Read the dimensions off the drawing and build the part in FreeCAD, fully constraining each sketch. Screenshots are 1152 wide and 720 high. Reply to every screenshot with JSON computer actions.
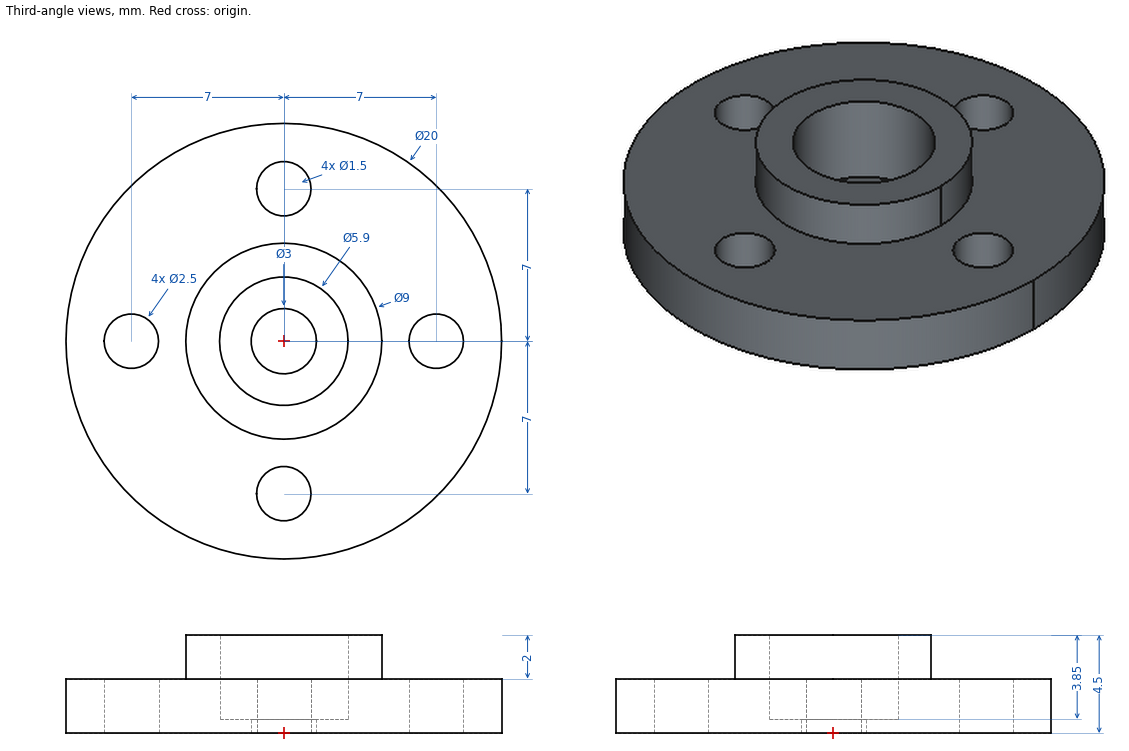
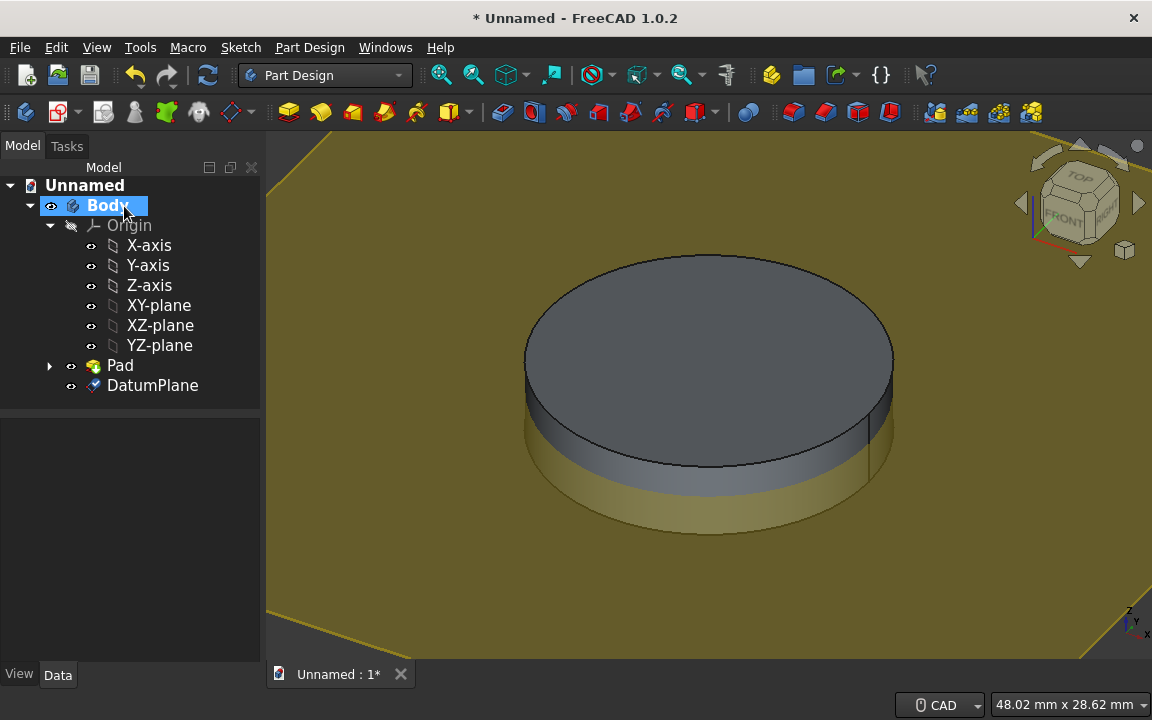
{"action": "left_click", "coordinate": [116, 386]}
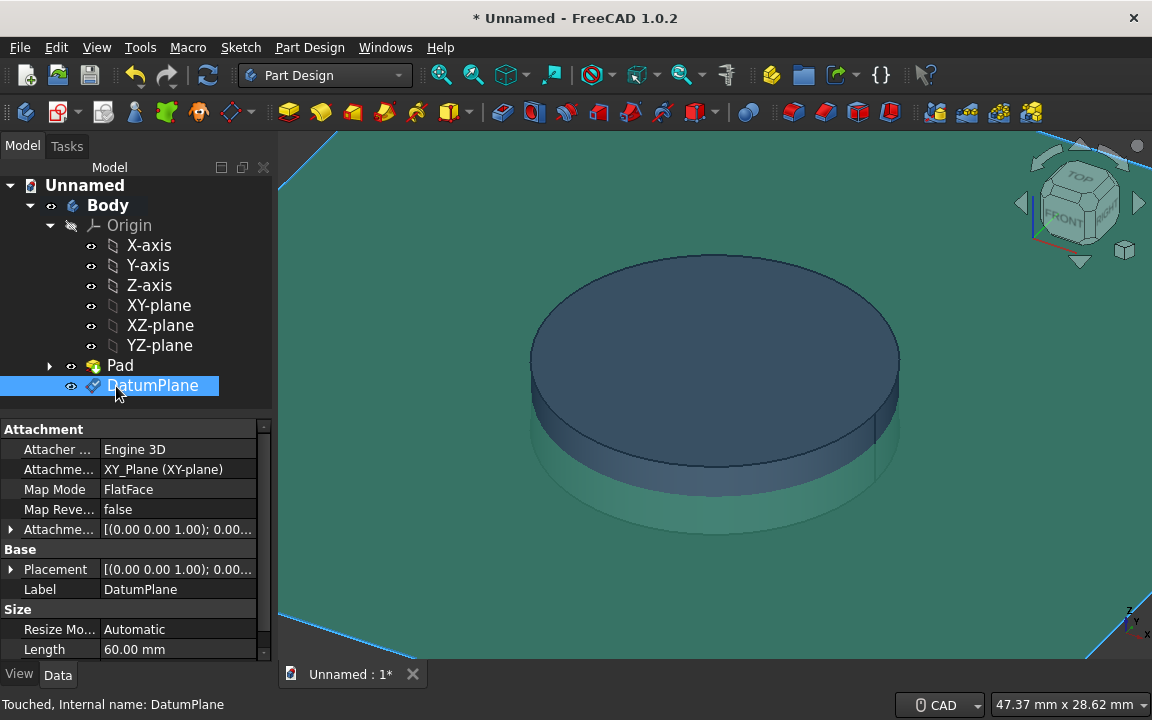
{"action": "left_click", "coordinate": [58, 112]}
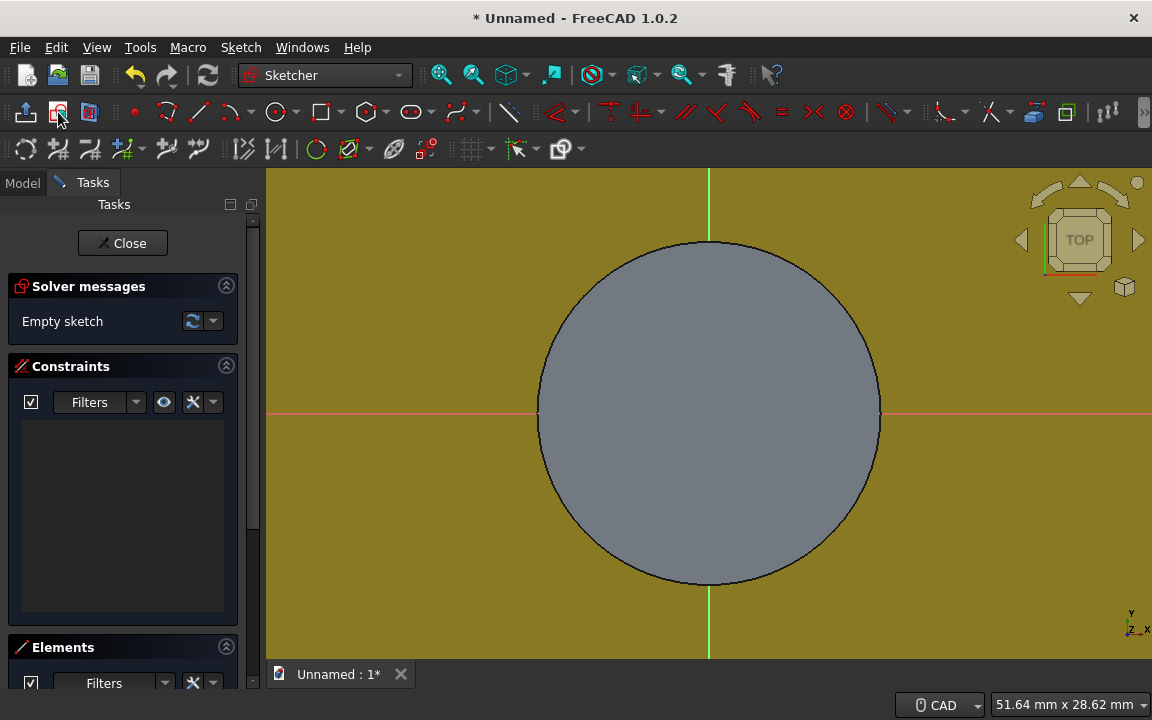
{"action": "key", "text": "q s"}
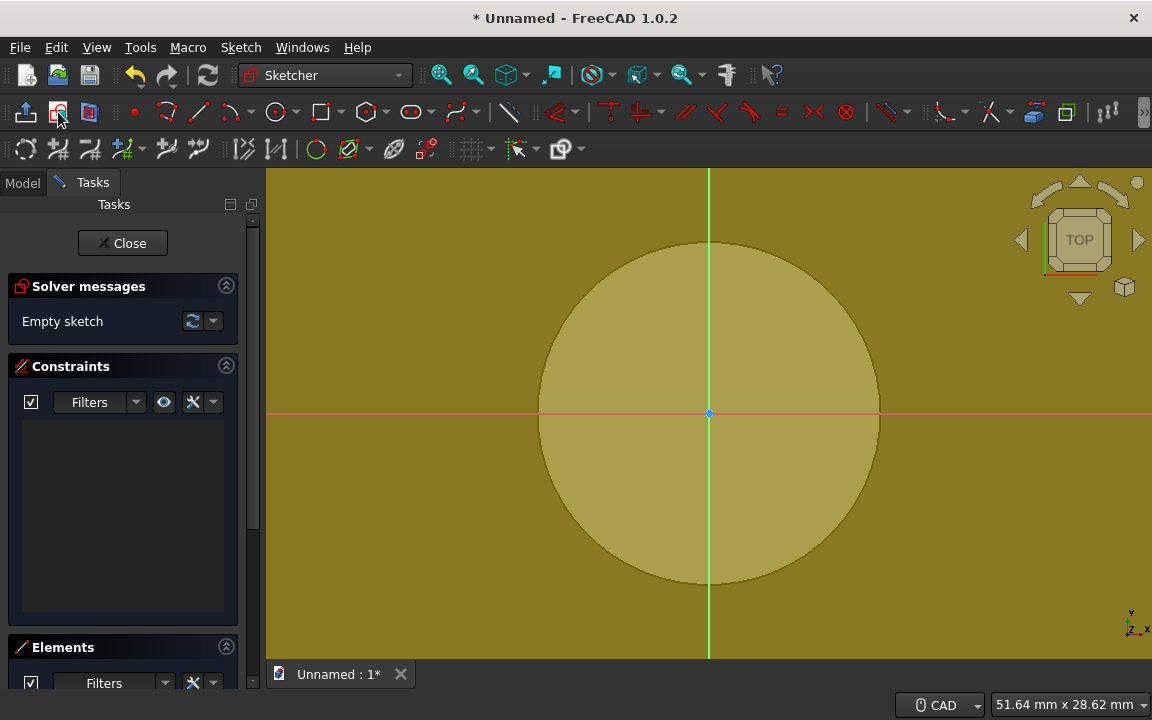
{"action": "key", "text": "g c"}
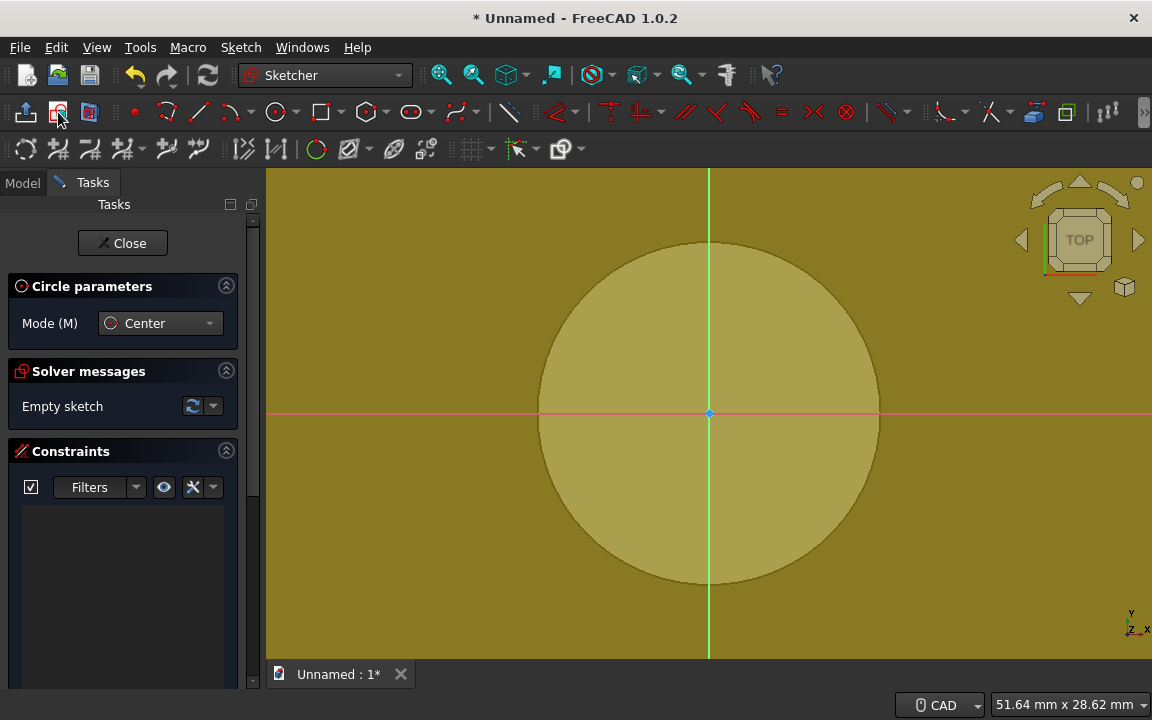
{"action": "left_click", "coordinate": [709, 414]}
{"action": "left_click", "coordinate": [830, 292]}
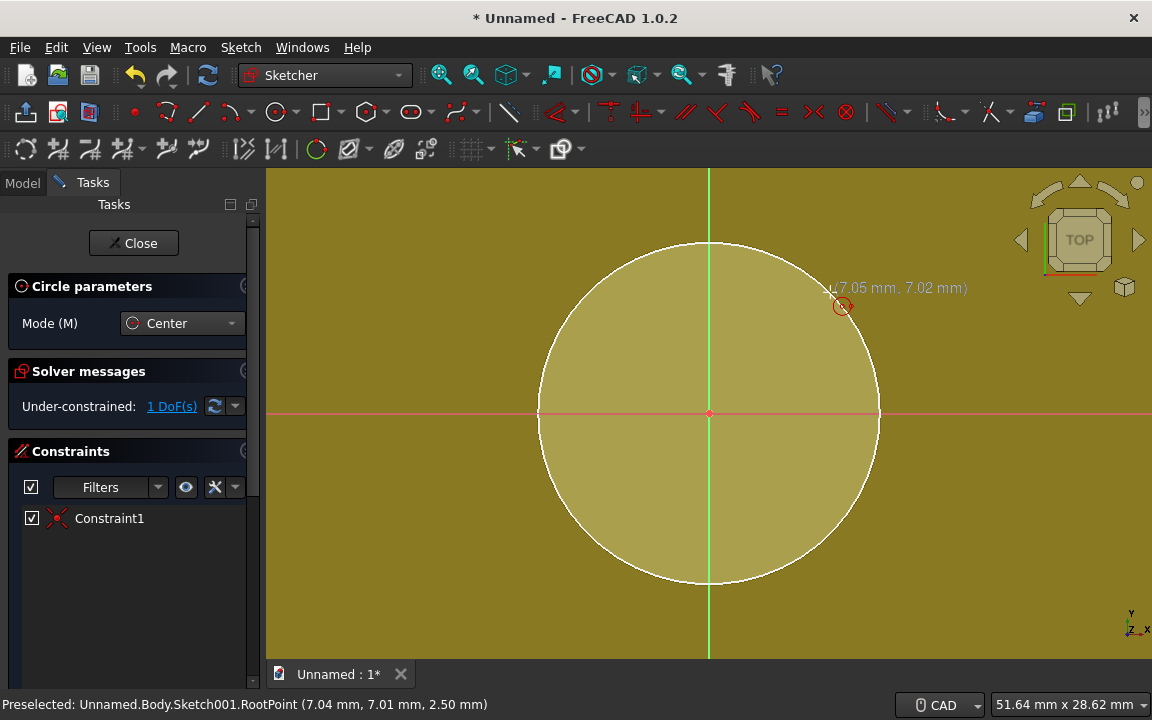
{"action": "left_click", "coordinate": [709, 414]}
{"action": "left_click", "coordinate": [764, 359]}
{"action": "key", "text": "Escape"}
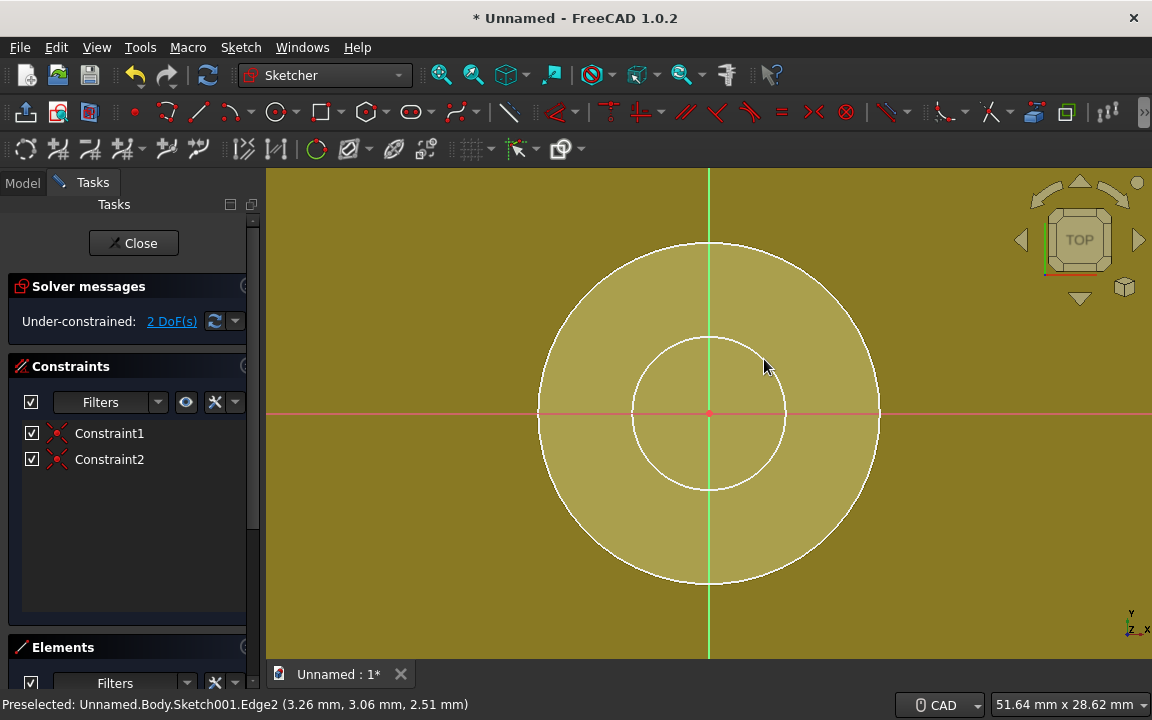
{"action": "left_click", "coordinate": [556, 112]}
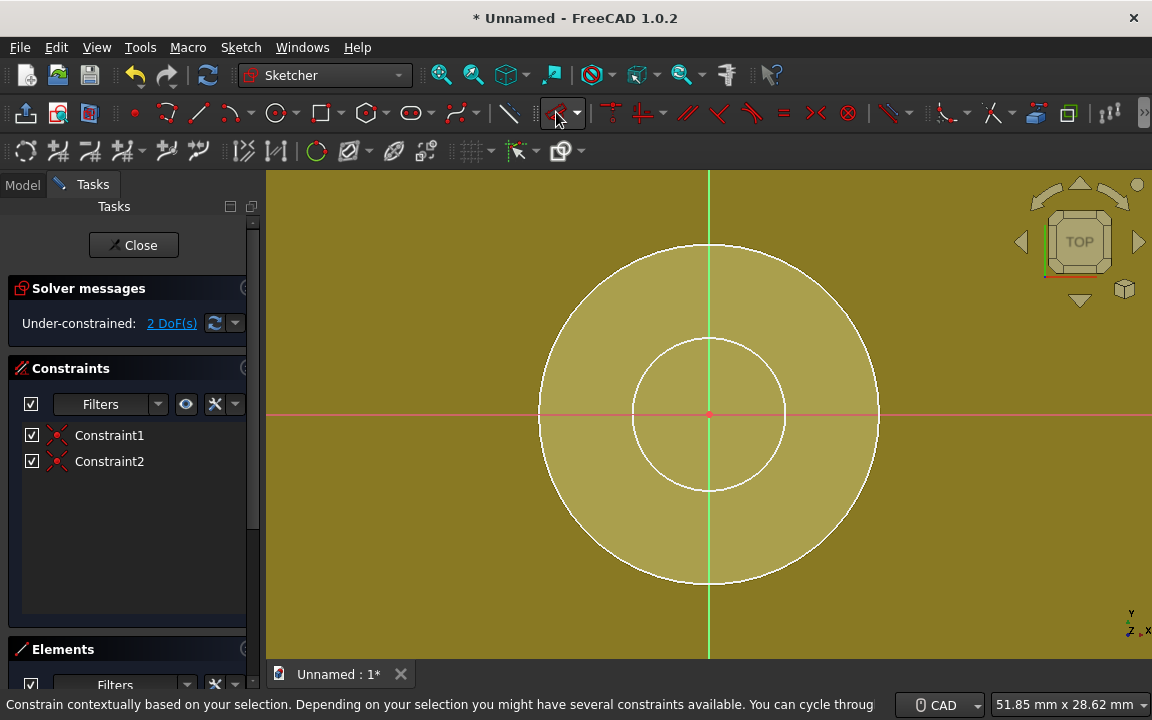
{"action": "left_click", "coordinate": [829, 294]}
{"action": "left_click", "coordinate": [852, 271]}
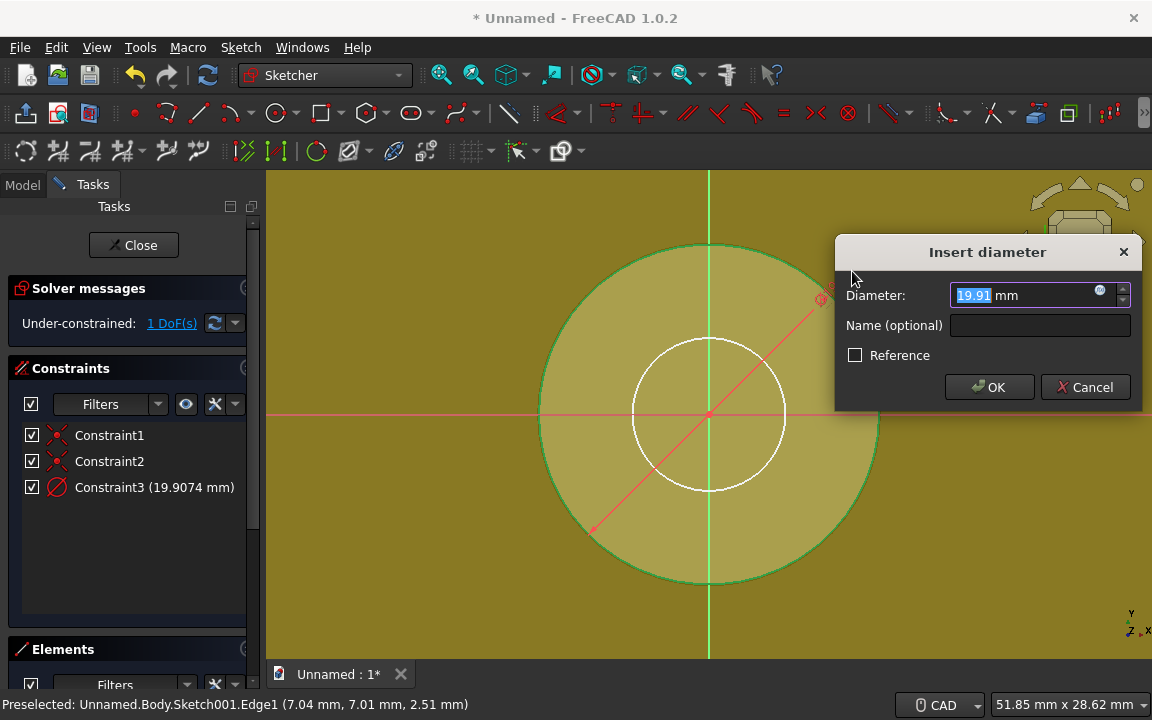
{"action": "type", "text": "20"}
{"action": "key", "text": "Return"}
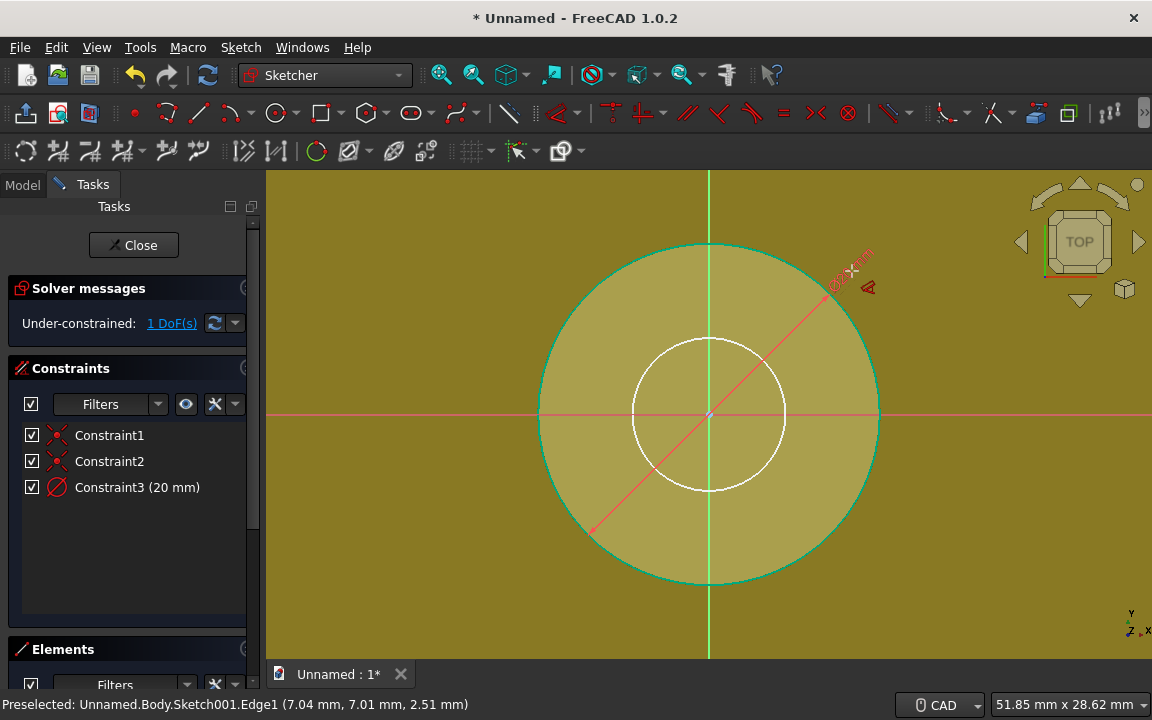
{"action": "left_click", "coordinate": [763, 360]}
{"action": "left_click", "coordinate": [786, 337]}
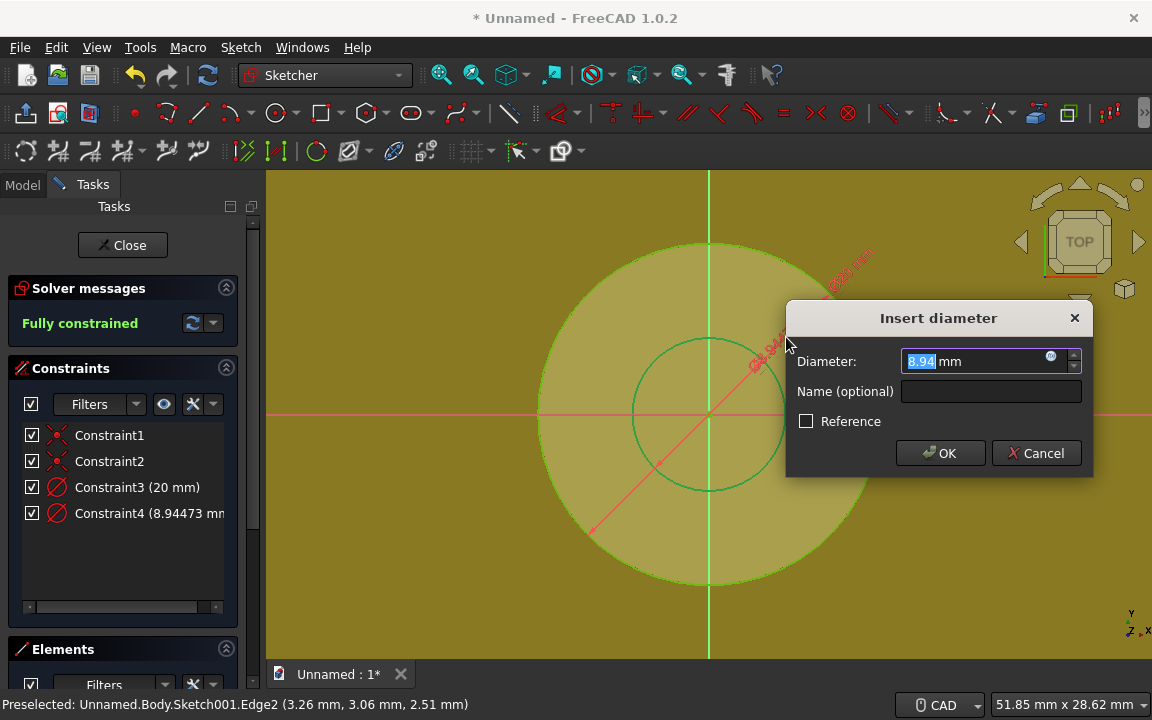
{"action": "type", "text": "9"}
{"action": "key", "text": "Return"}
{"action": "key", "text": "Escape"}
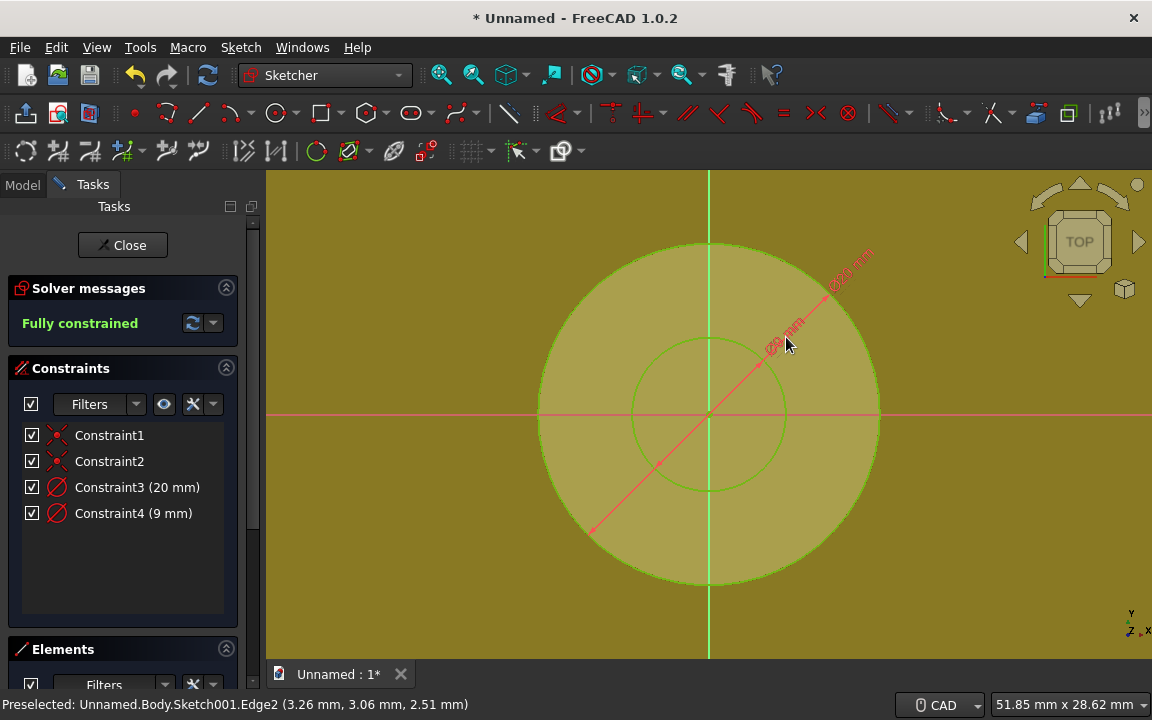
{"action": "left_click", "coordinate": [123, 245]}